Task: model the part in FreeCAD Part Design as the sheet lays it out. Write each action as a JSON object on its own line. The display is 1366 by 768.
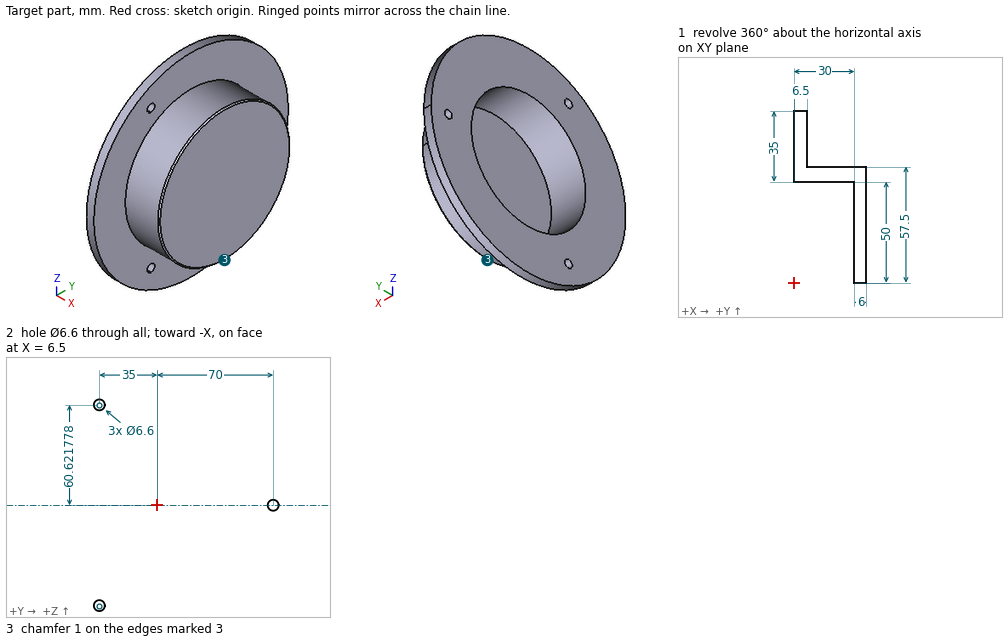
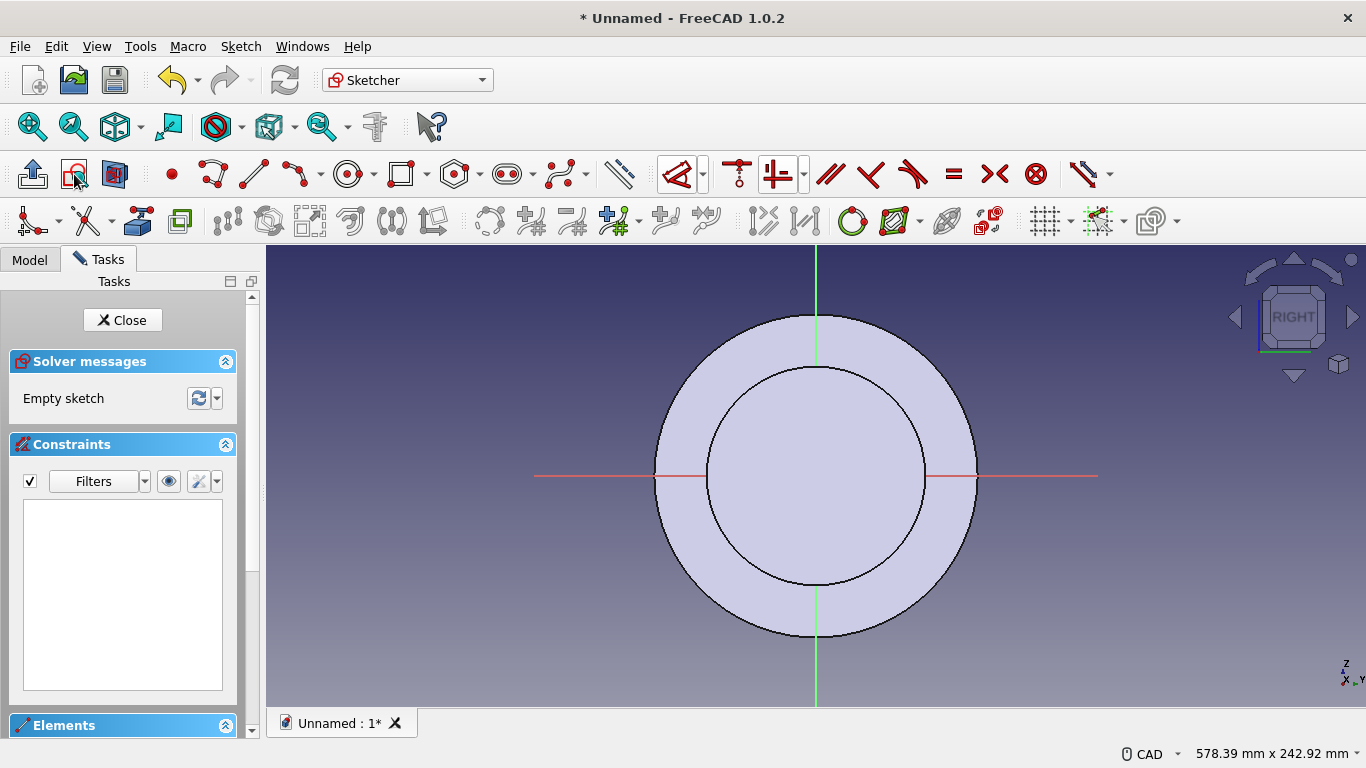
{"action": "left_click", "coordinate": [115, 174]}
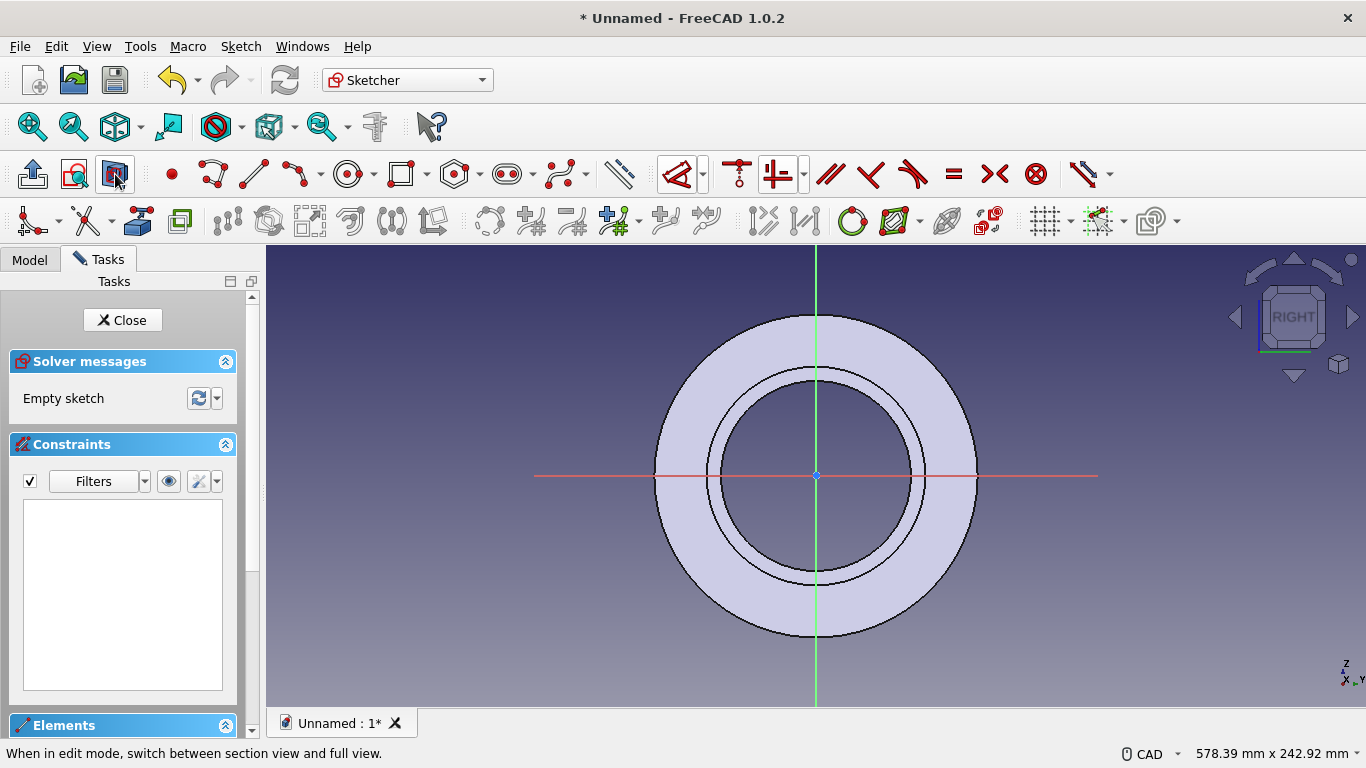
{"action": "left_click", "coordinate": [348, 174]}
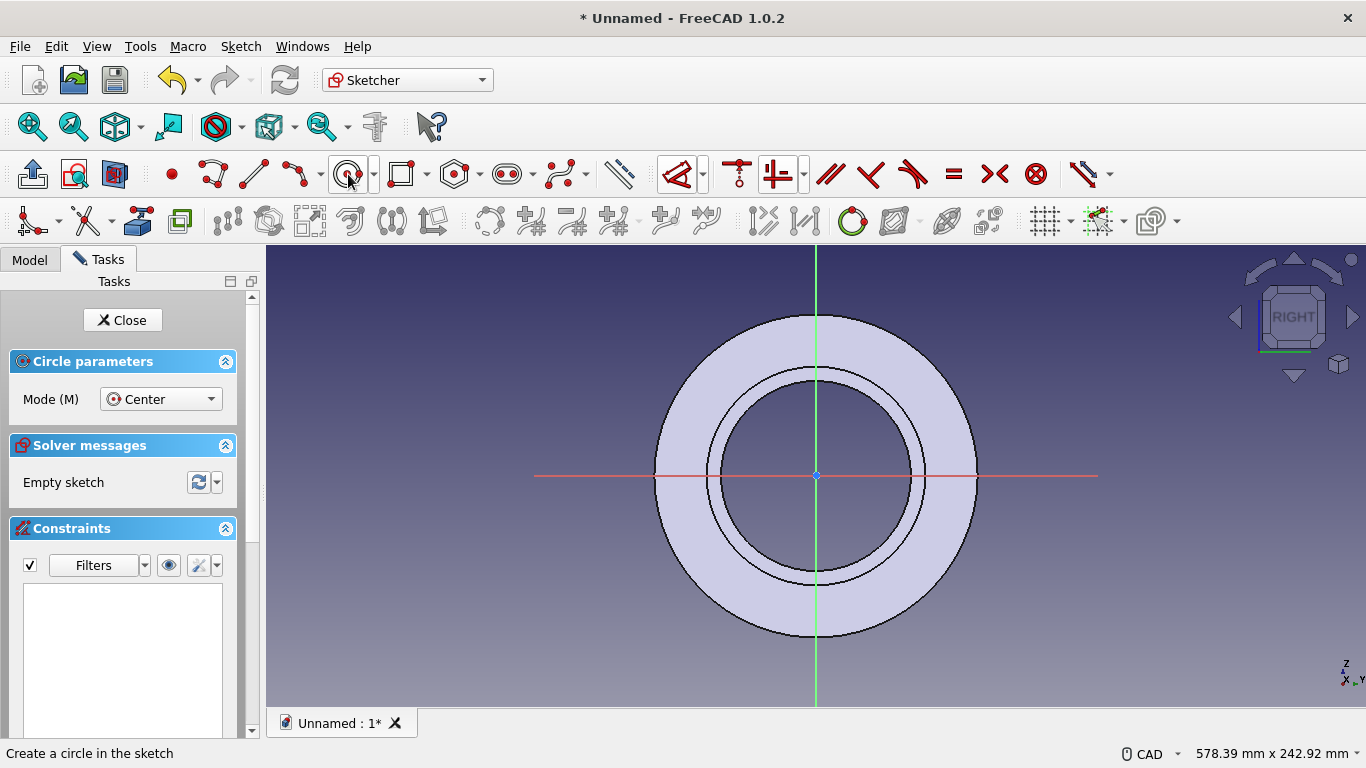
{"action": "scroll", "coordinate": [749, 361], "scroll_direction": "up", "scroll_amount": 7}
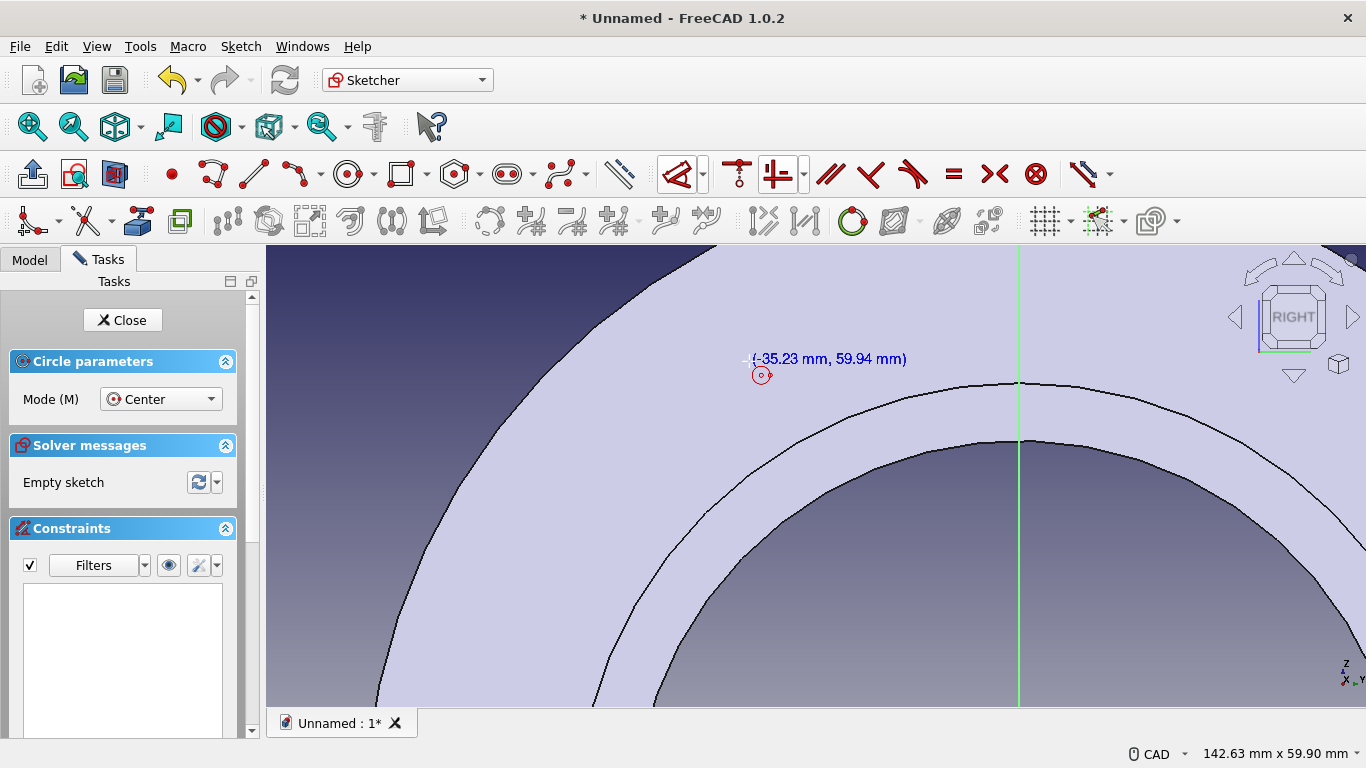
{"action": "scroll", "coordinate": [572, 325], "scroll_direction": "down", "scroll_amount": 6}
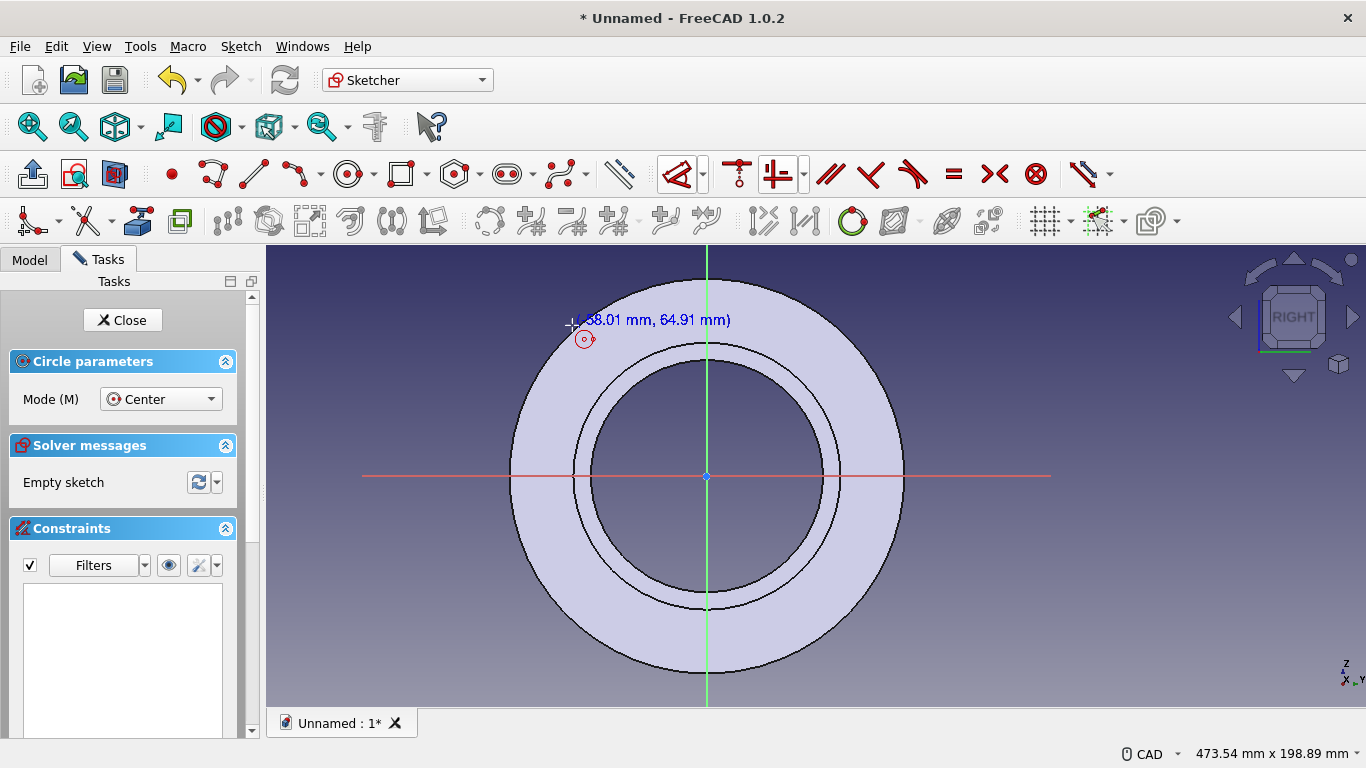
{"action": "left_click", "coordinate": [626, 335]}
{"action": "mouse_move", "coordinate": [631, 330]}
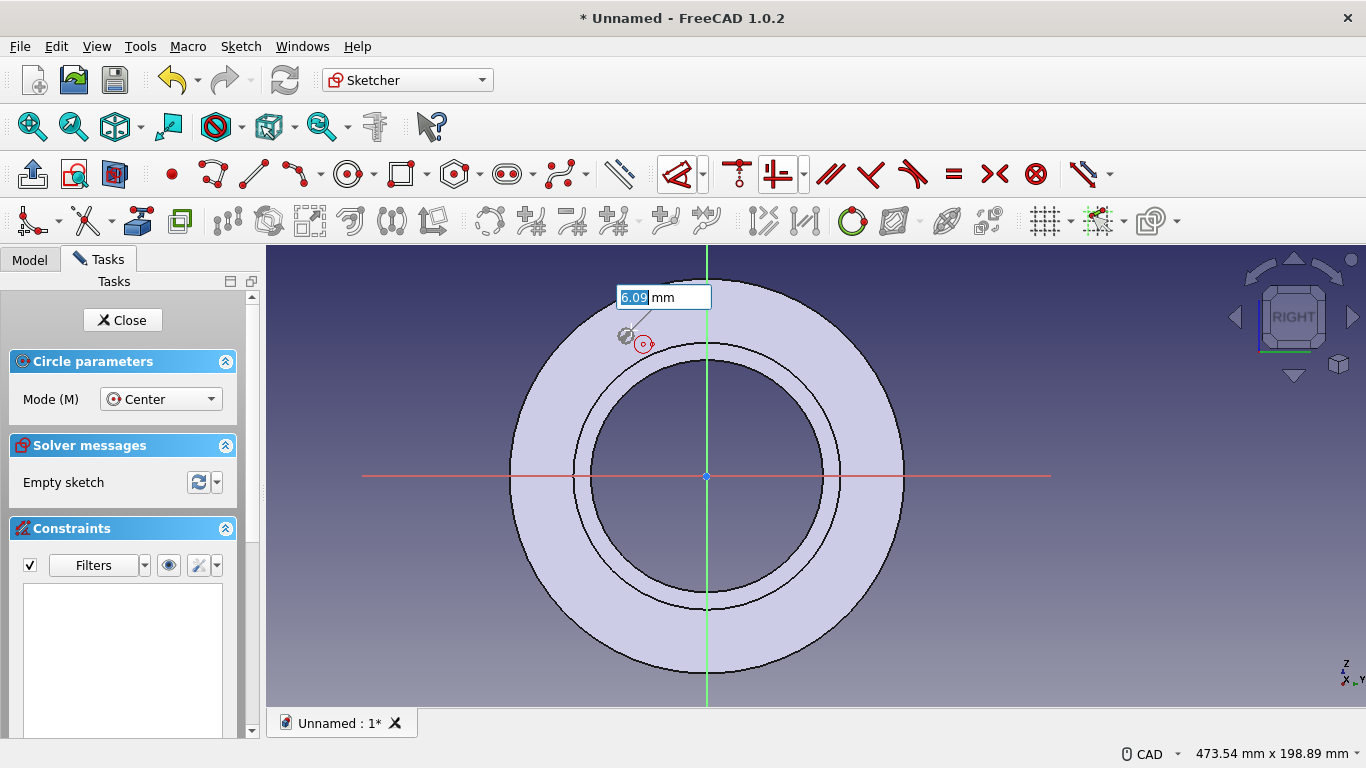
{"action": "type", "text": "6.6"}
{"action": "key", "text": "Return"}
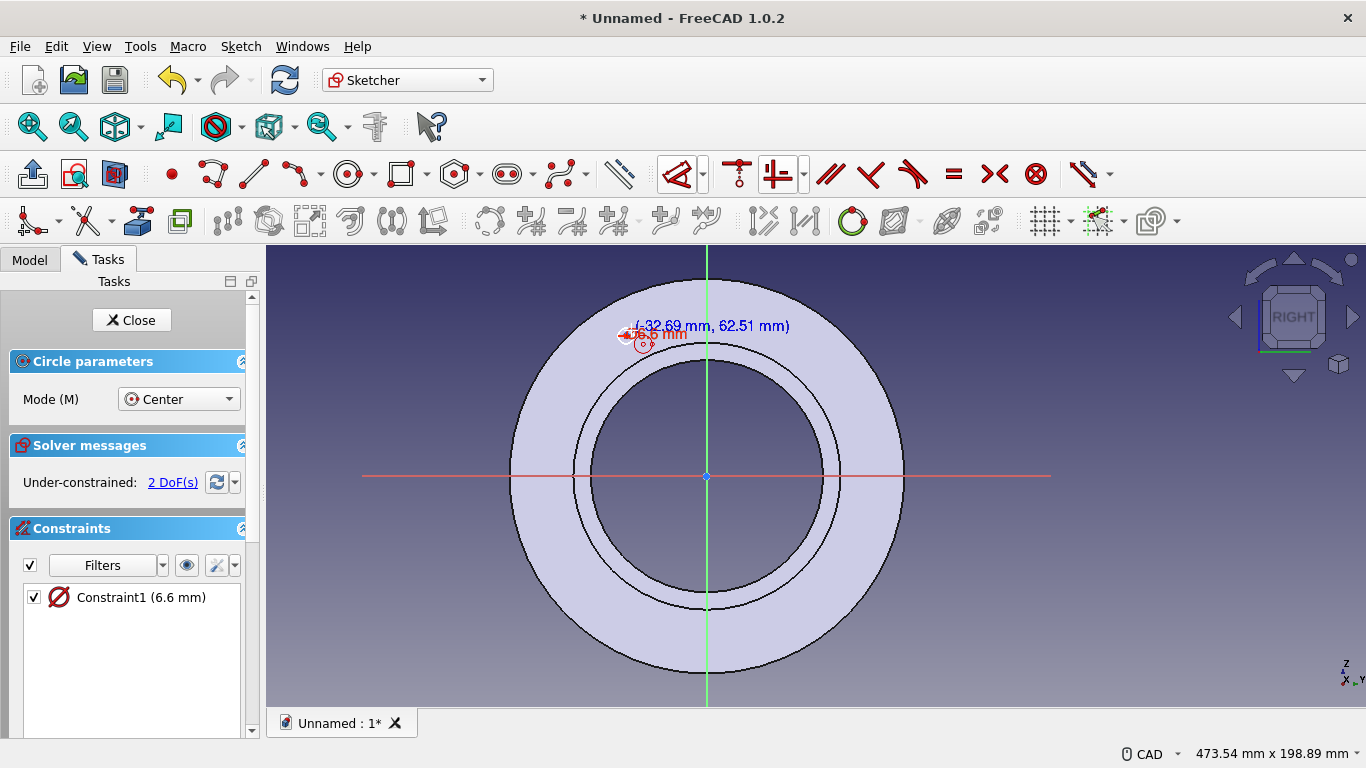
{"action": "scroll", "coordinate": [870, 476], "scroll_direction": "up", "scroll_amount": 6}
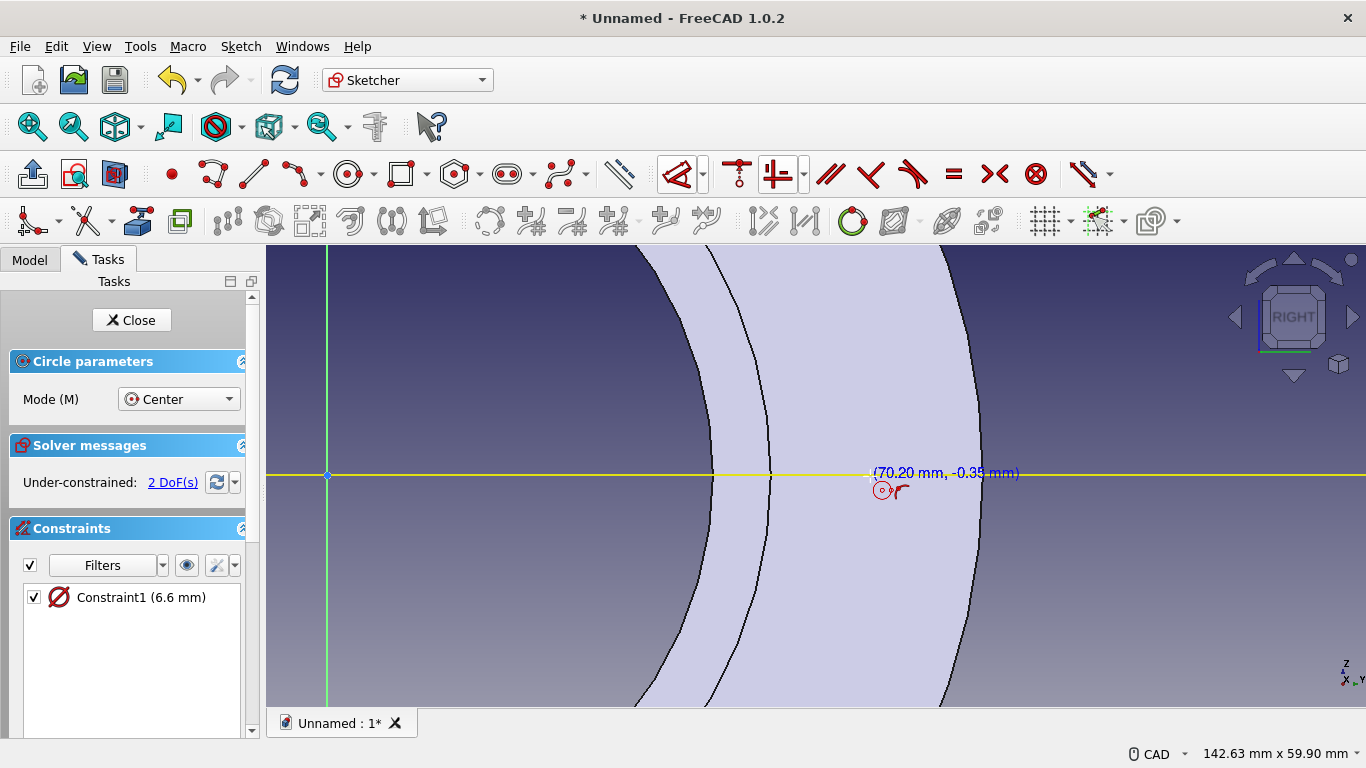
{"action": "scroll", "coordinate": [870, 476], "scroll_direction": "down", "scroll_amount": 6}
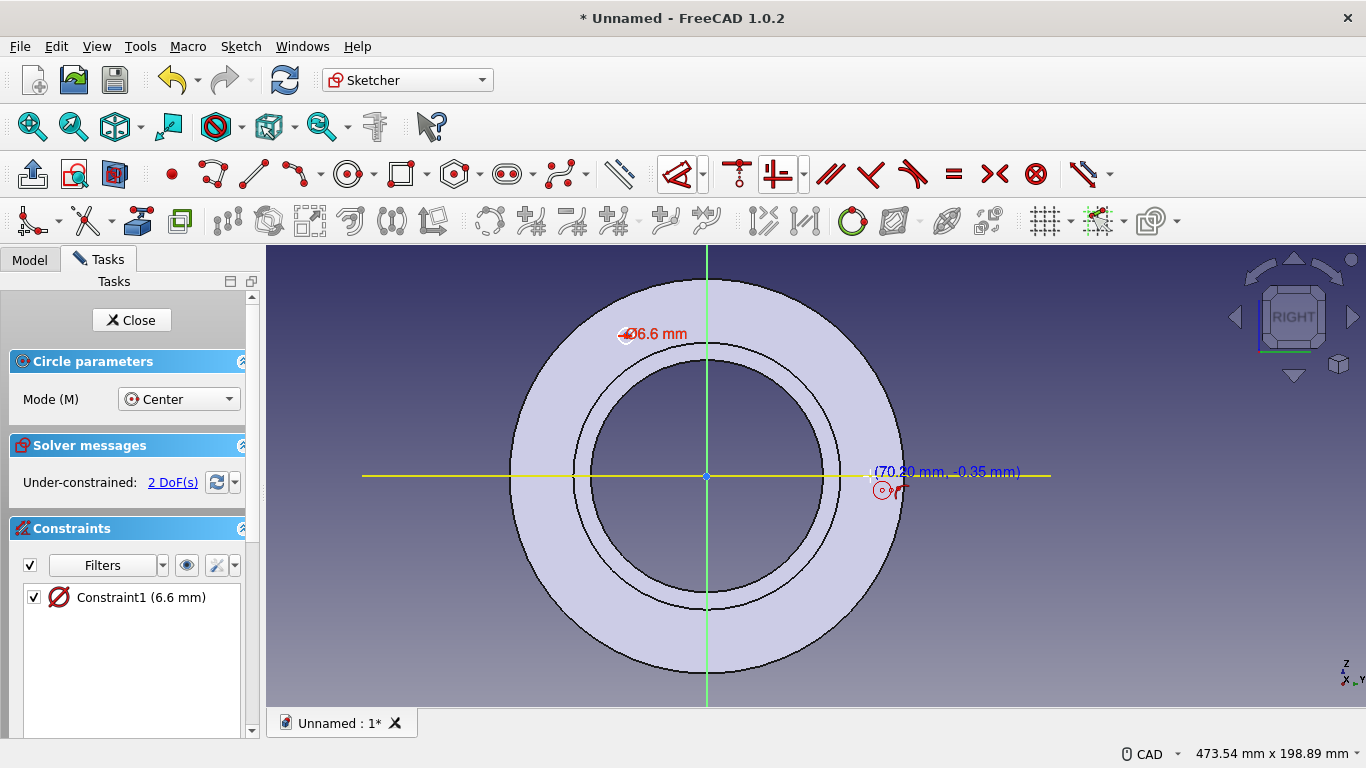
{"action": "left_click", "coordinate": [870, 476]}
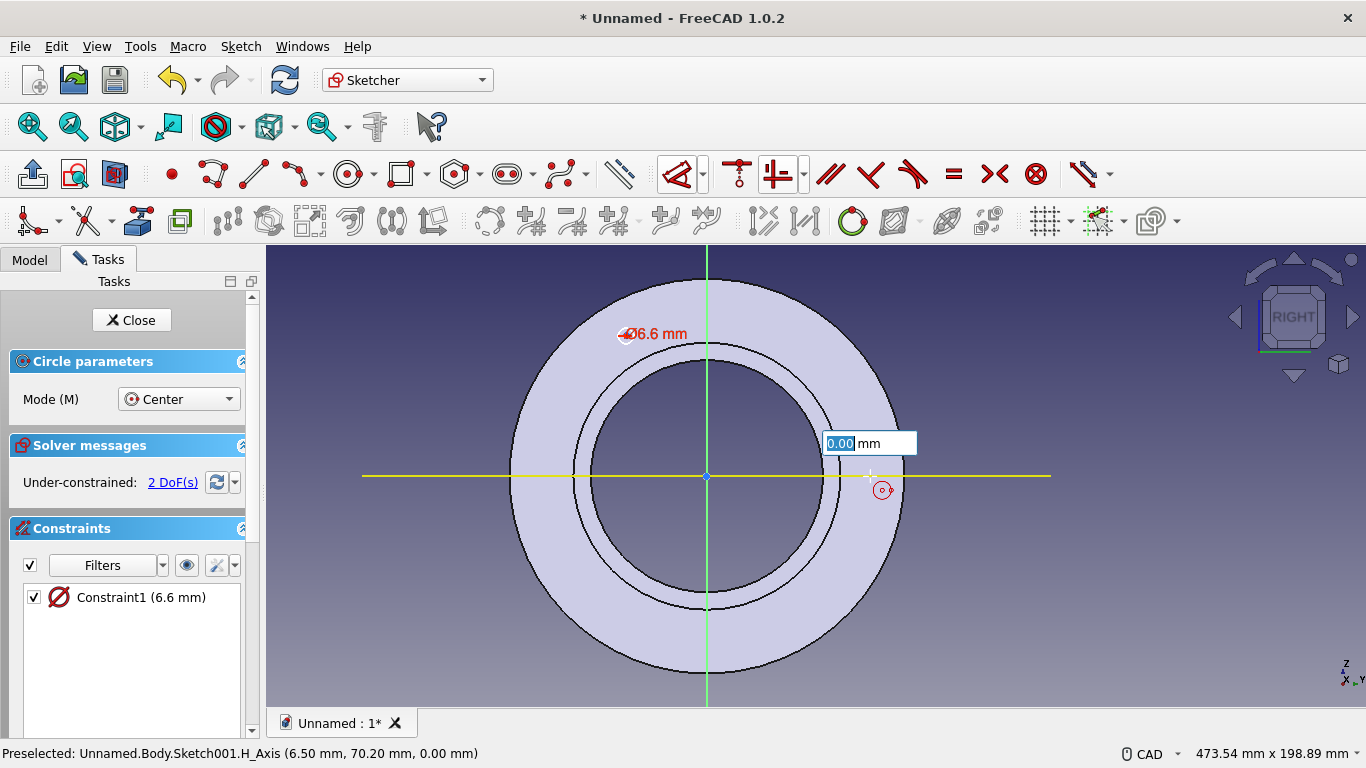
{"action": "scroll", "coordinate": [867, 483], "scroll_direction": "up", "scroll_amount": 4}
{"action": "mouse_move", "coordinate": [866, 483]}